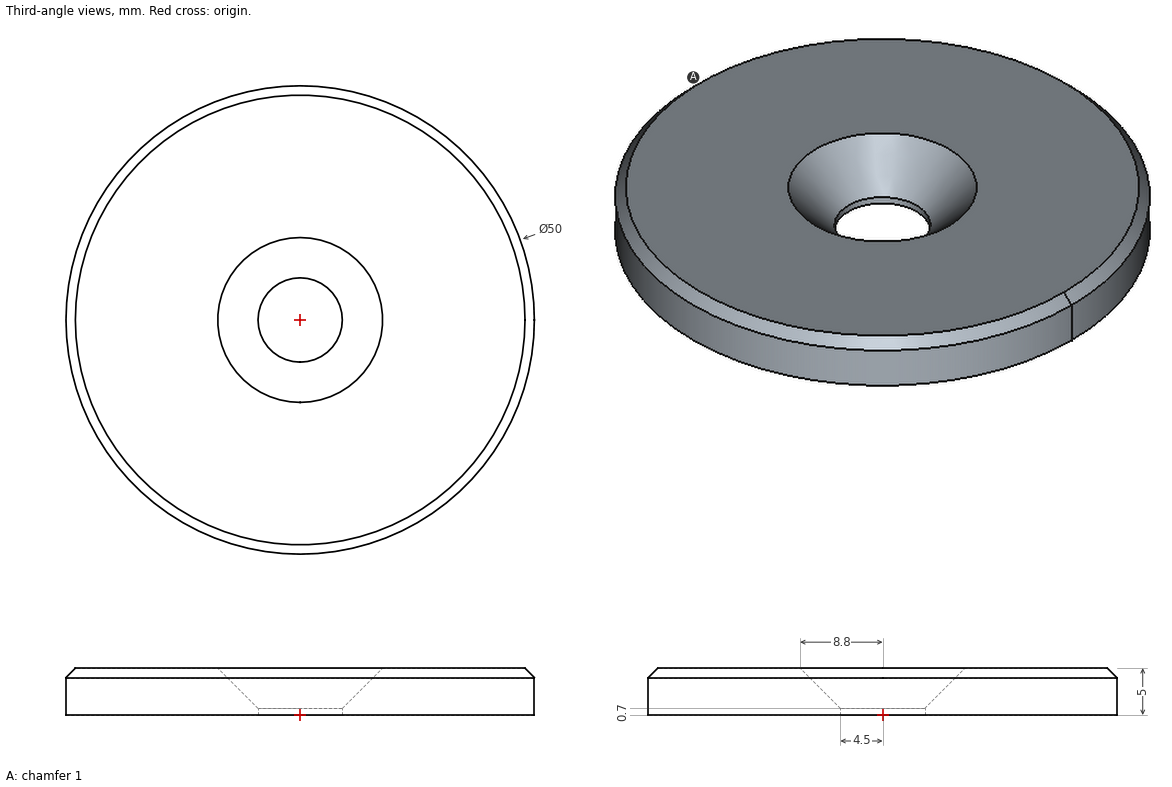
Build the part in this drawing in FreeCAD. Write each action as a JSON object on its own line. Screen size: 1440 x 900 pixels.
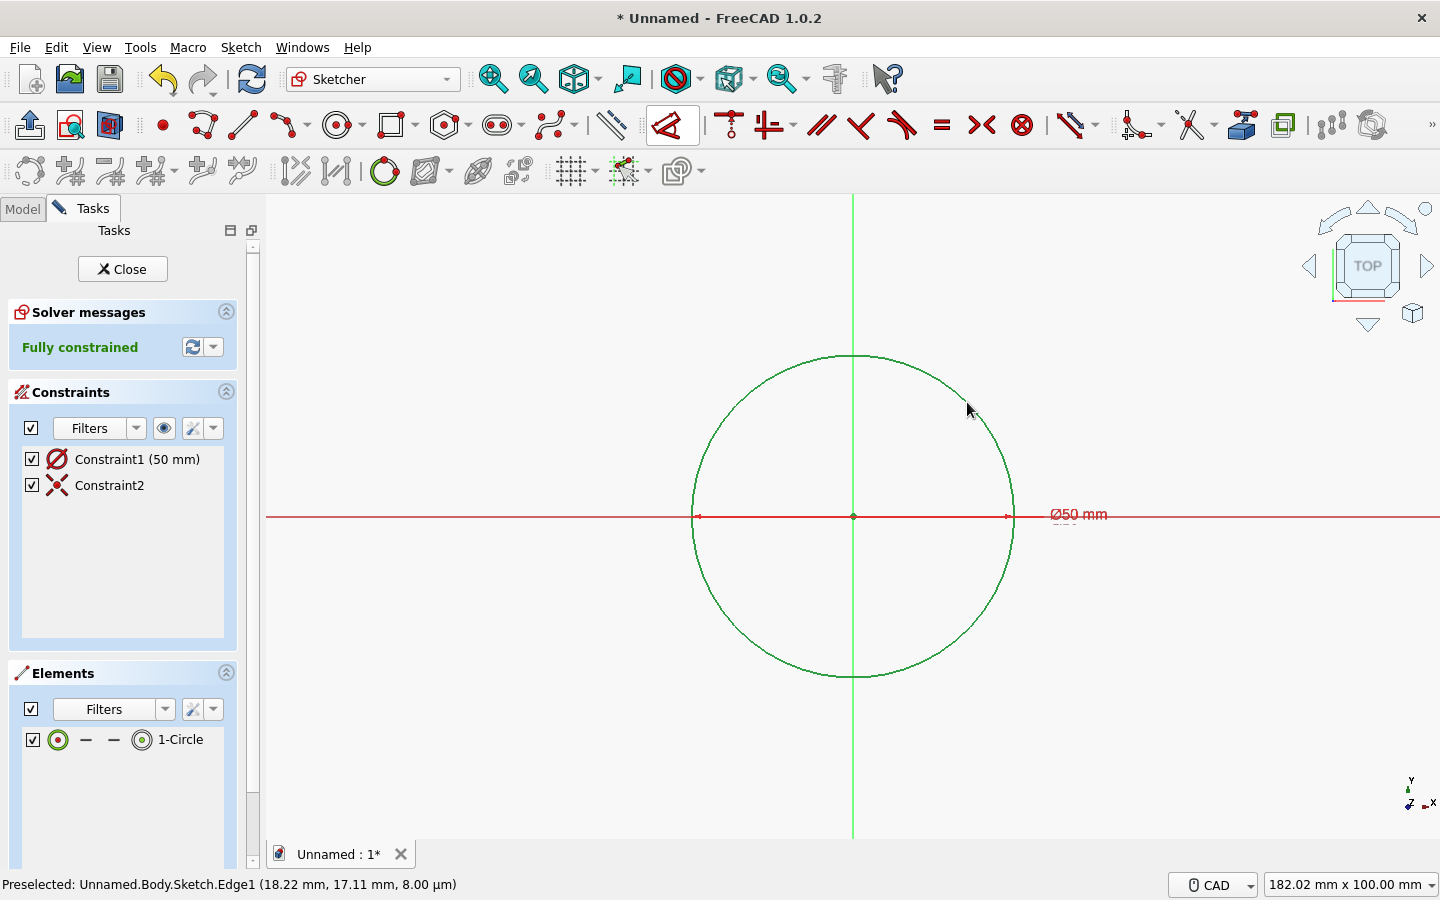
{"action": "left_click", "coordinate": [123, 269]}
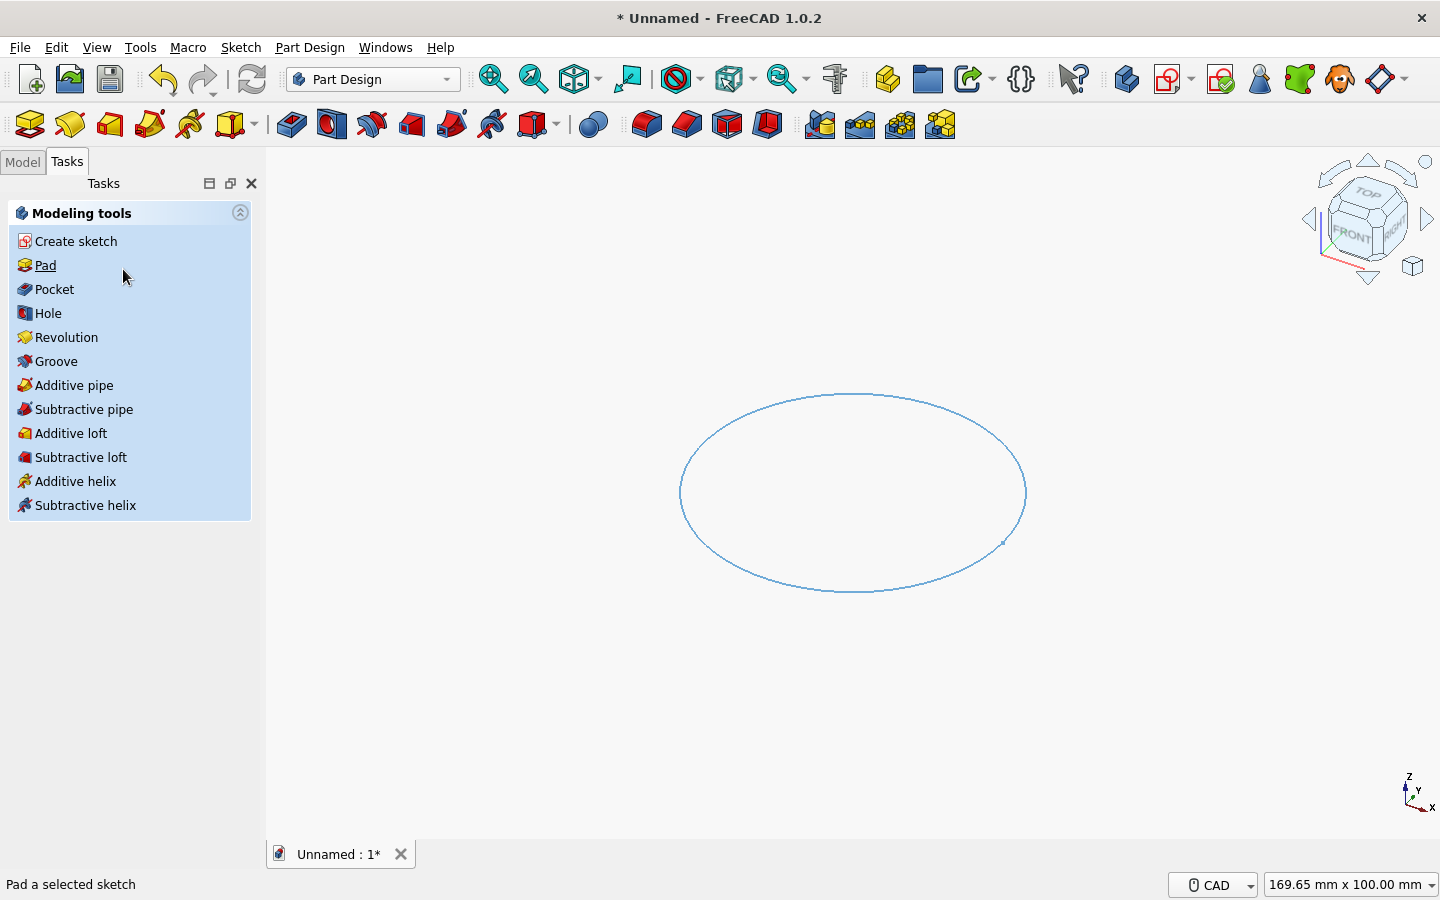
{"action": "left_click", "coordinate": [30, 124]}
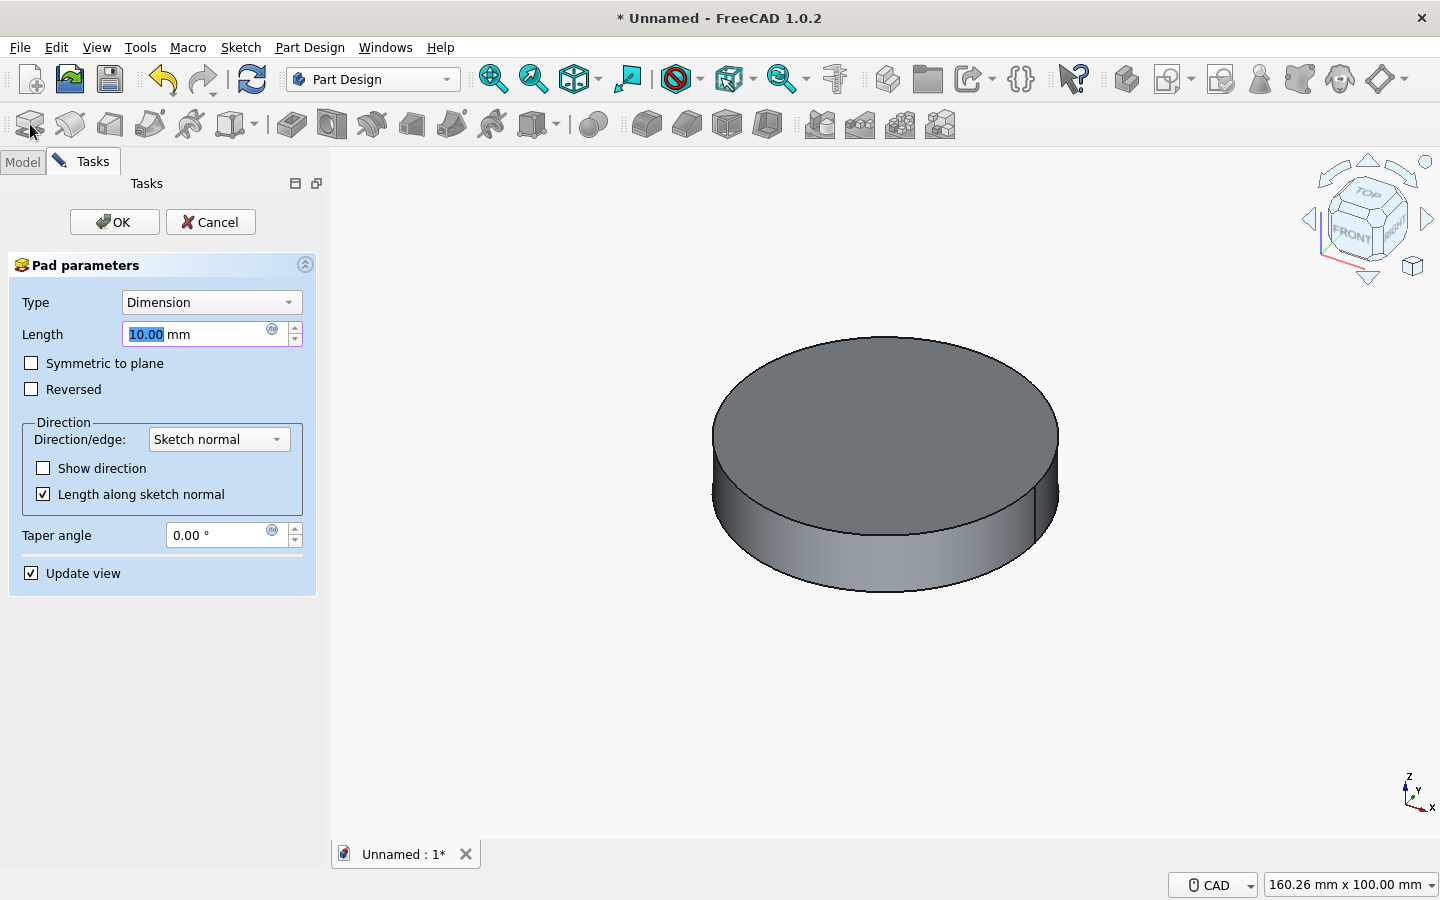
{"action": "type", "text": "5"}
{"action": "key", "text": "Tab"}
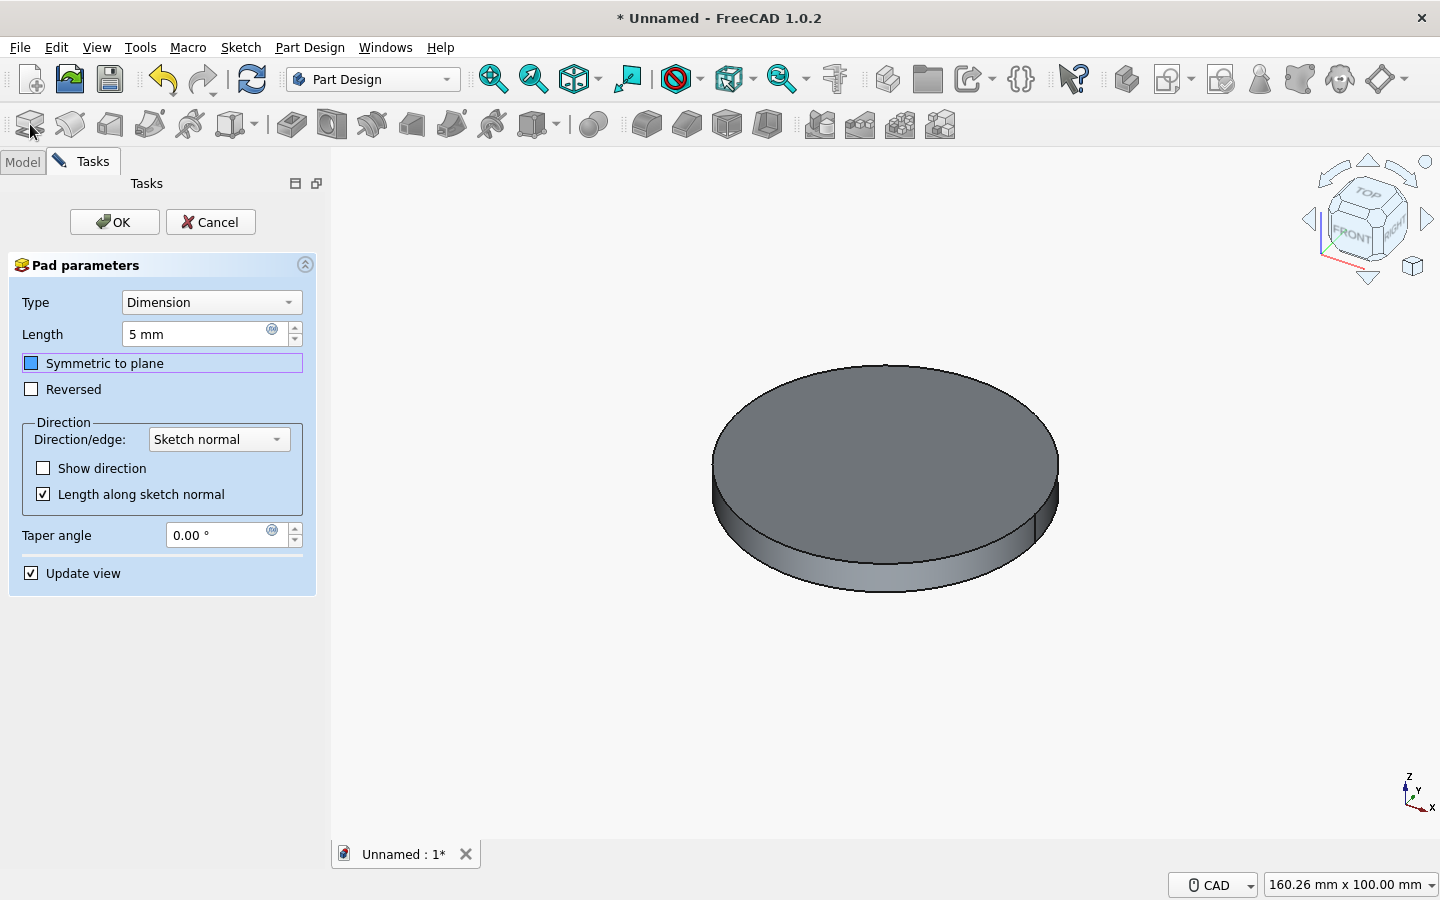
{"action": "left_click", "coordinate": [115, 222]}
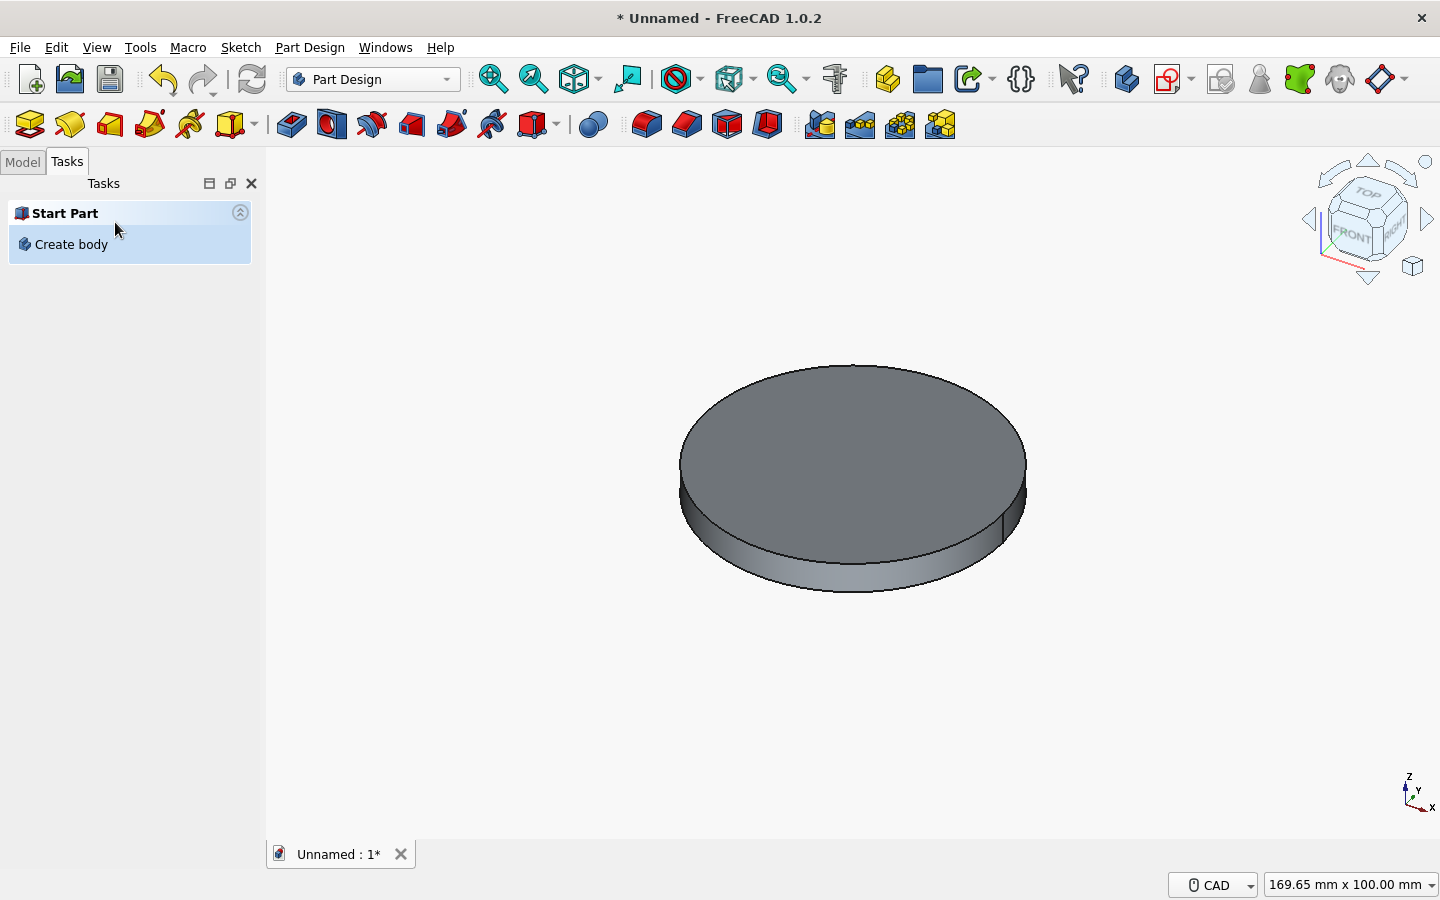
{"action": "left_click", "coordinate": [494, 80]}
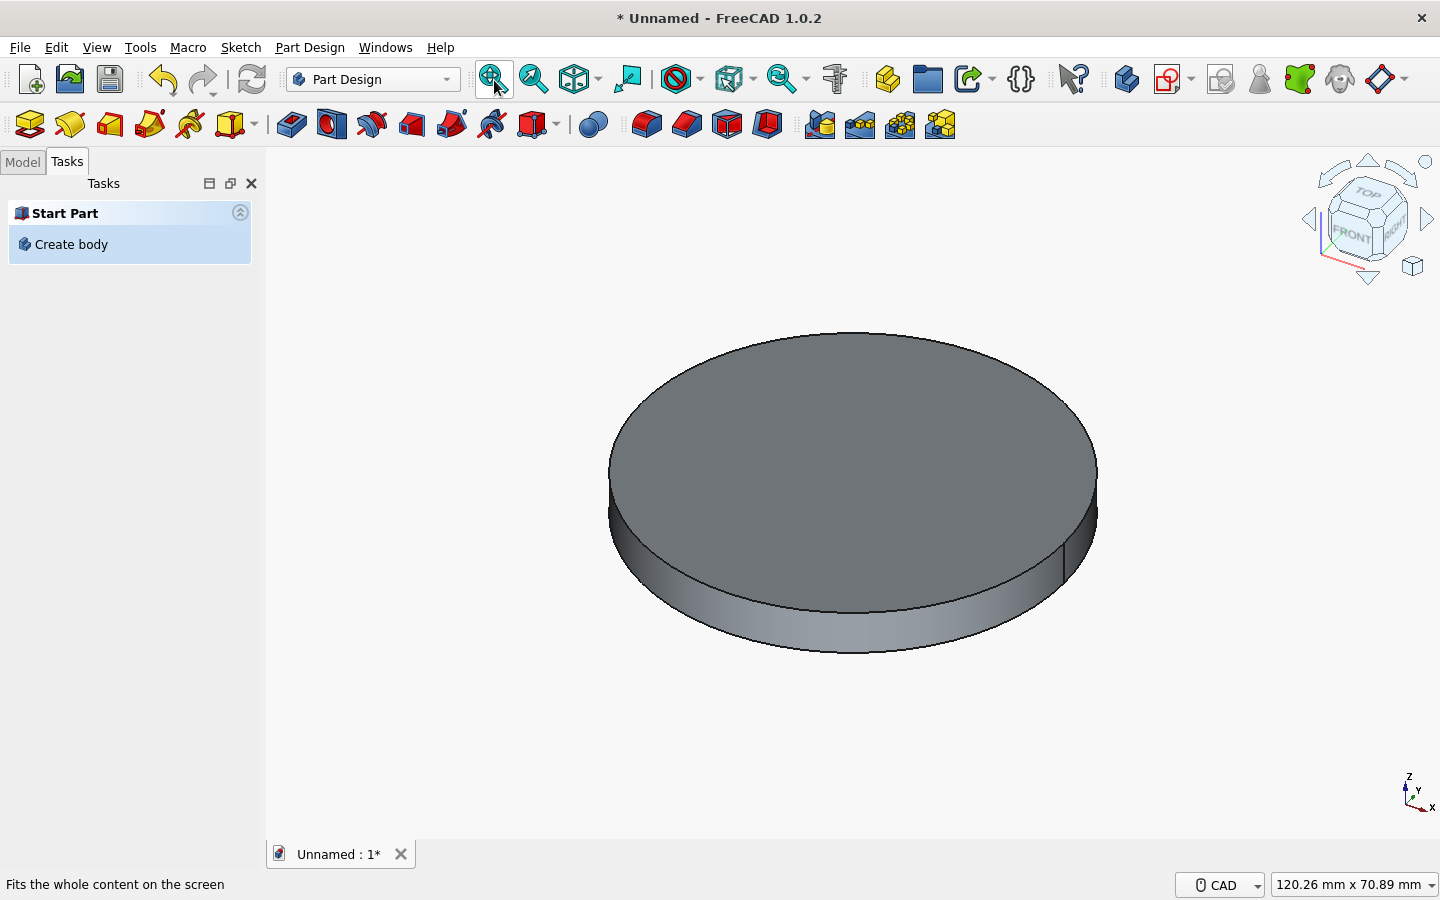
{"action": "left_click", "coordinate": [1168, 80]}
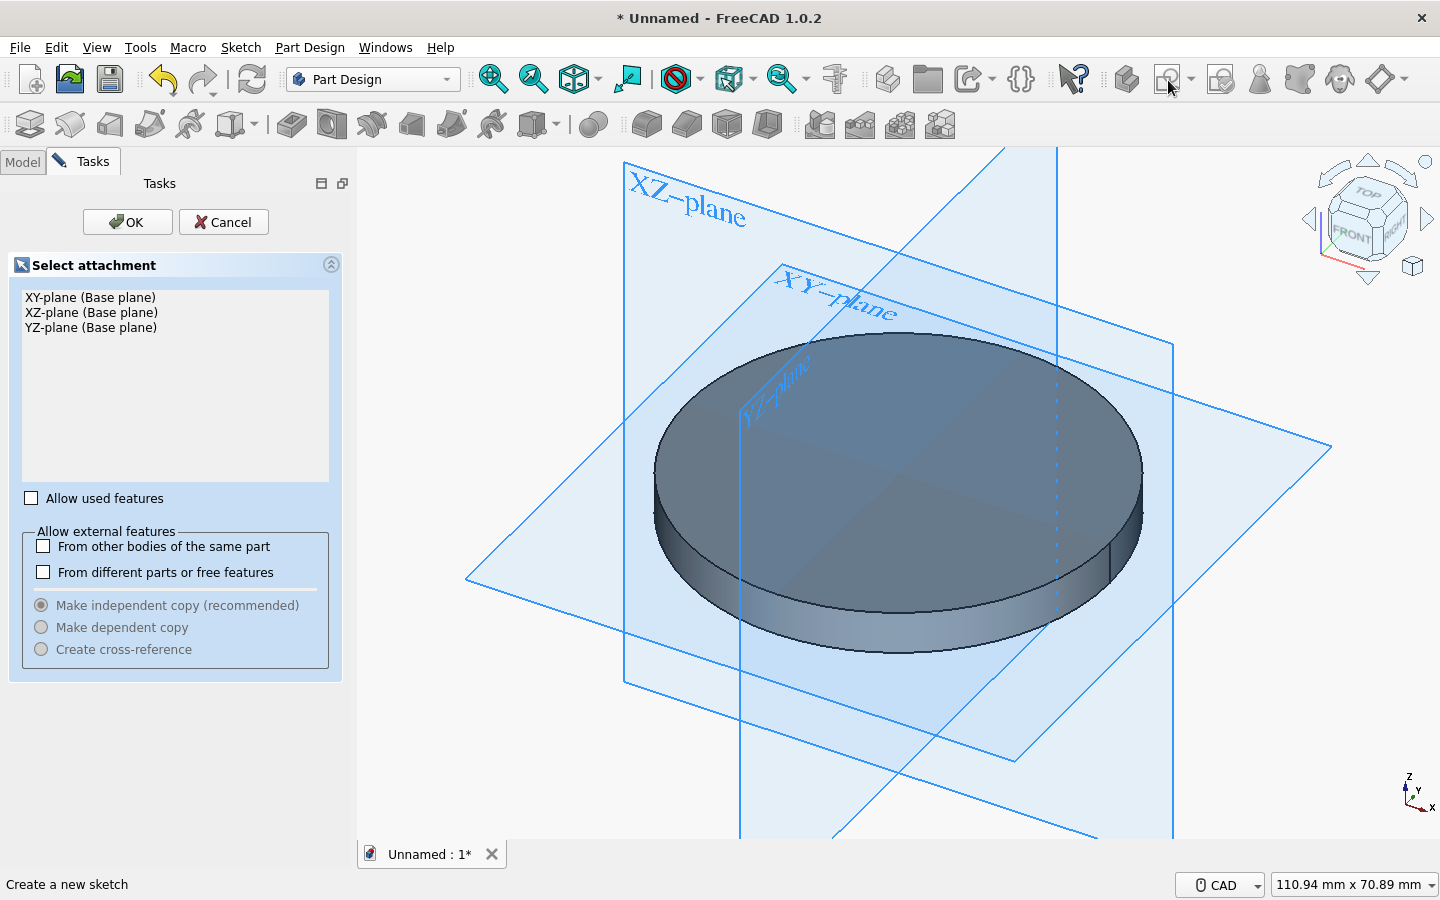
{"action": "left_click", "coordinate": [82, 328]}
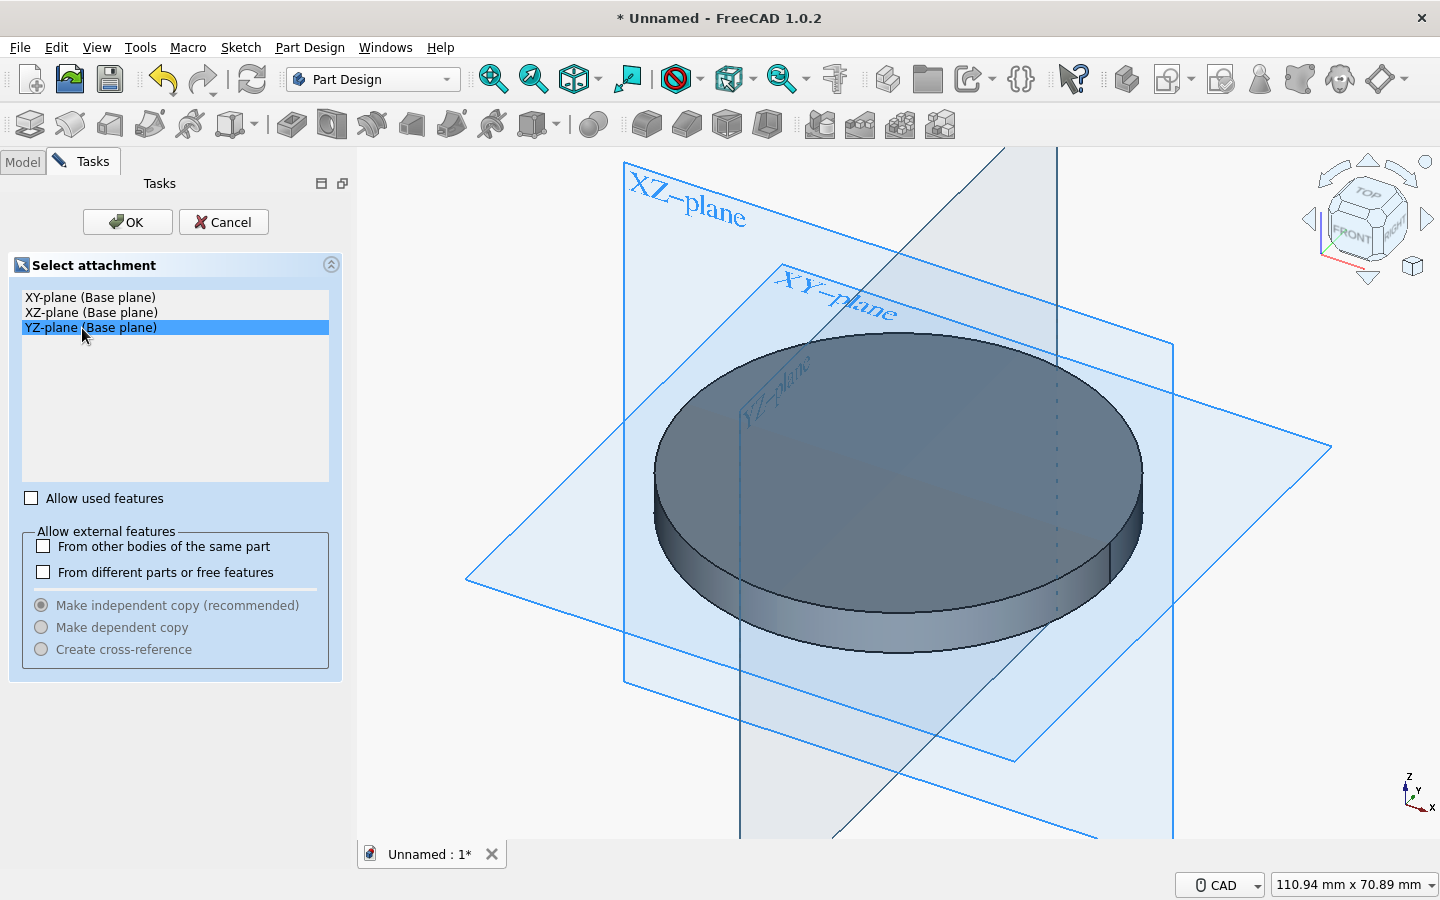
{"action": "left_click", "coordinate": [128, 222]}